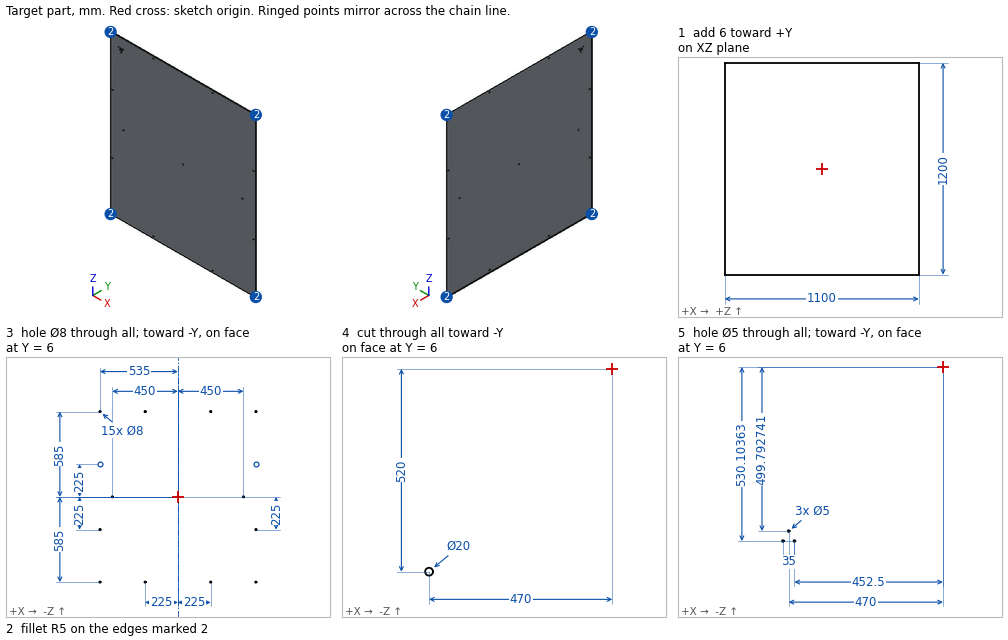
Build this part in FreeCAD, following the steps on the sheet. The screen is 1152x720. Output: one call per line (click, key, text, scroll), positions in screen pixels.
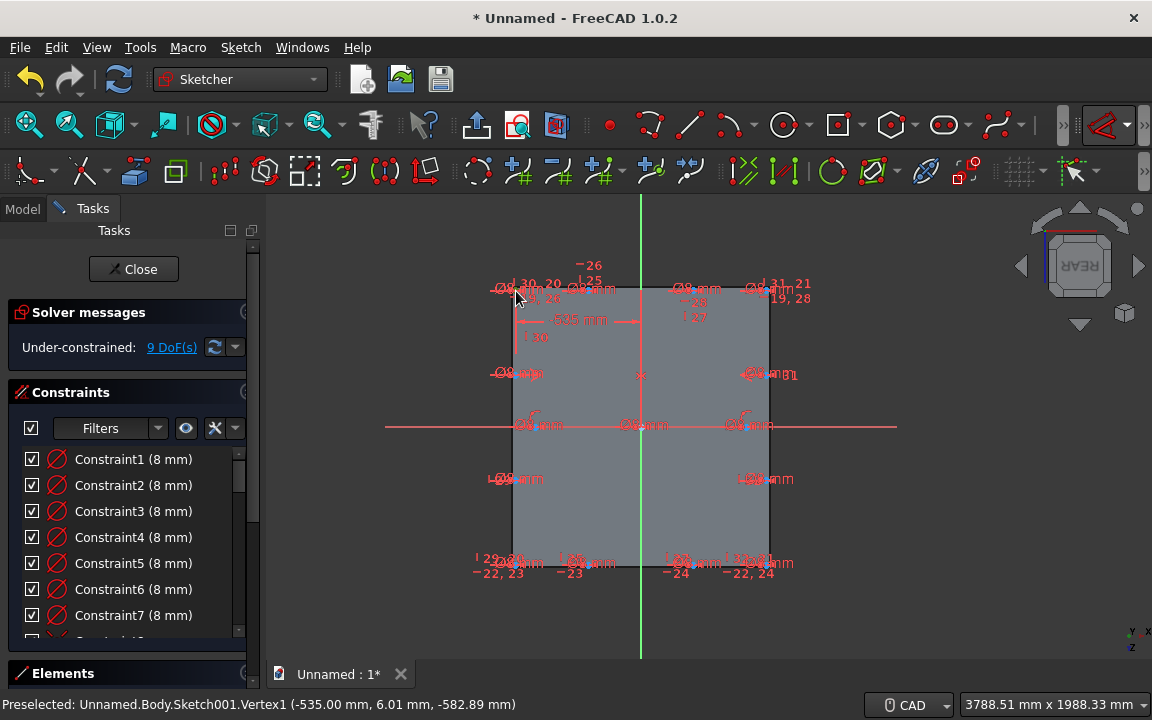
key(i)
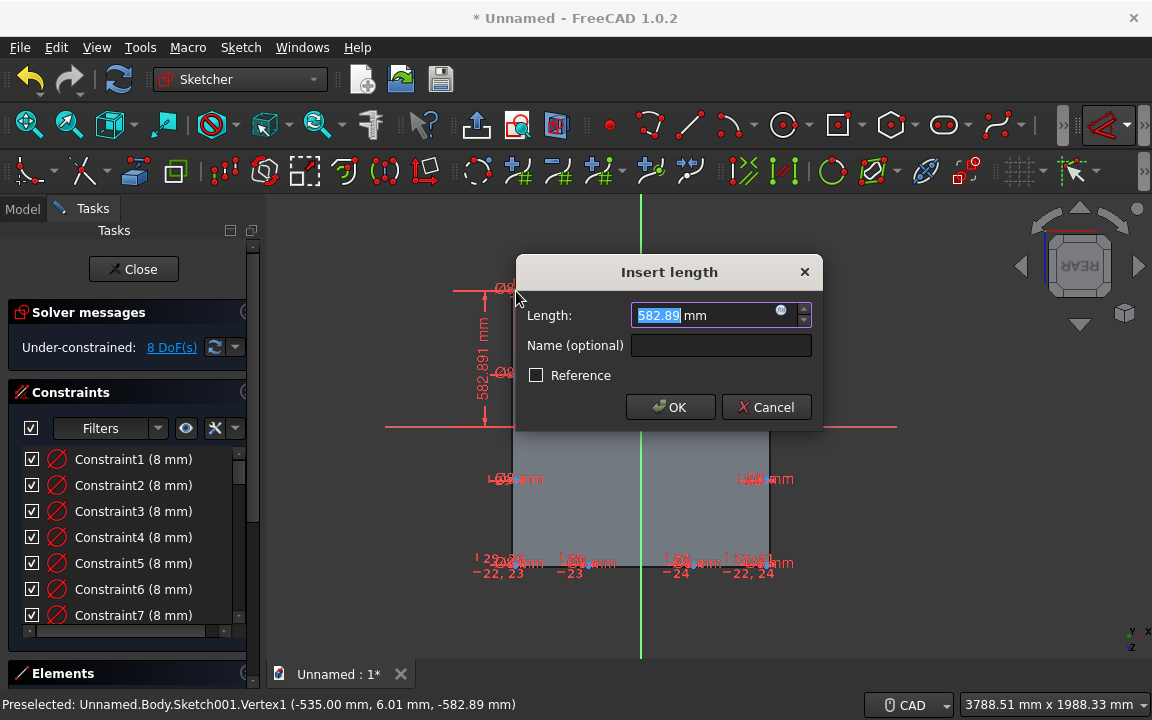
text(585)
key(Return)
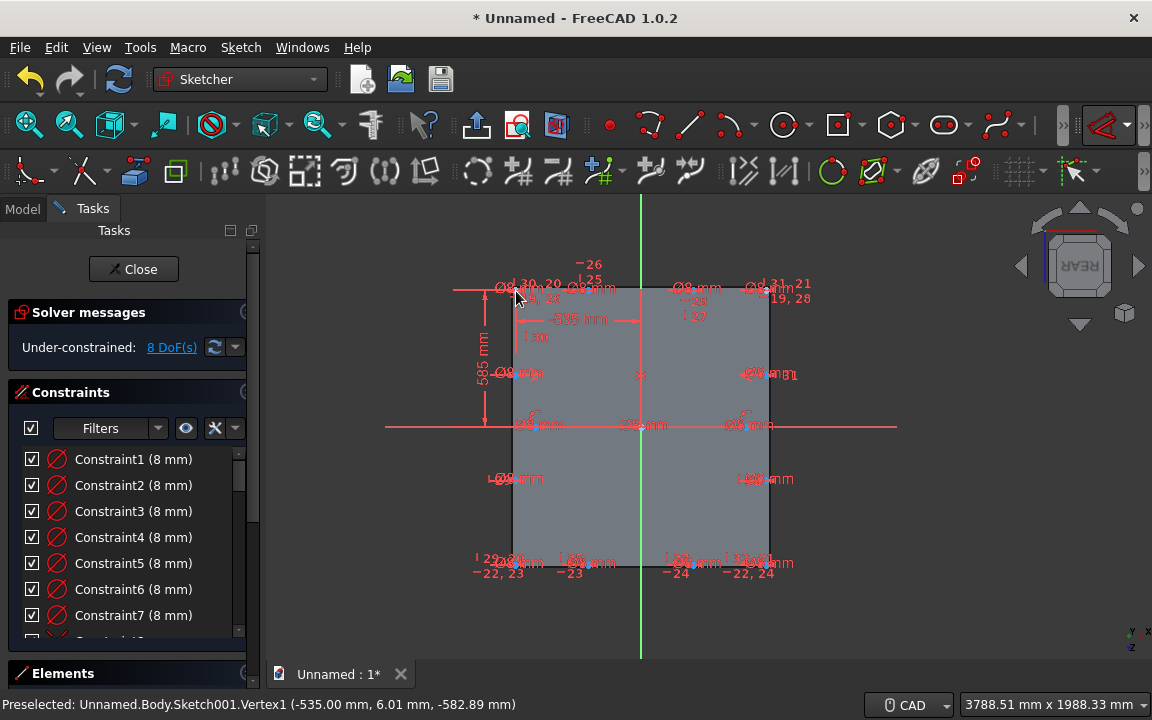
click(516, 565)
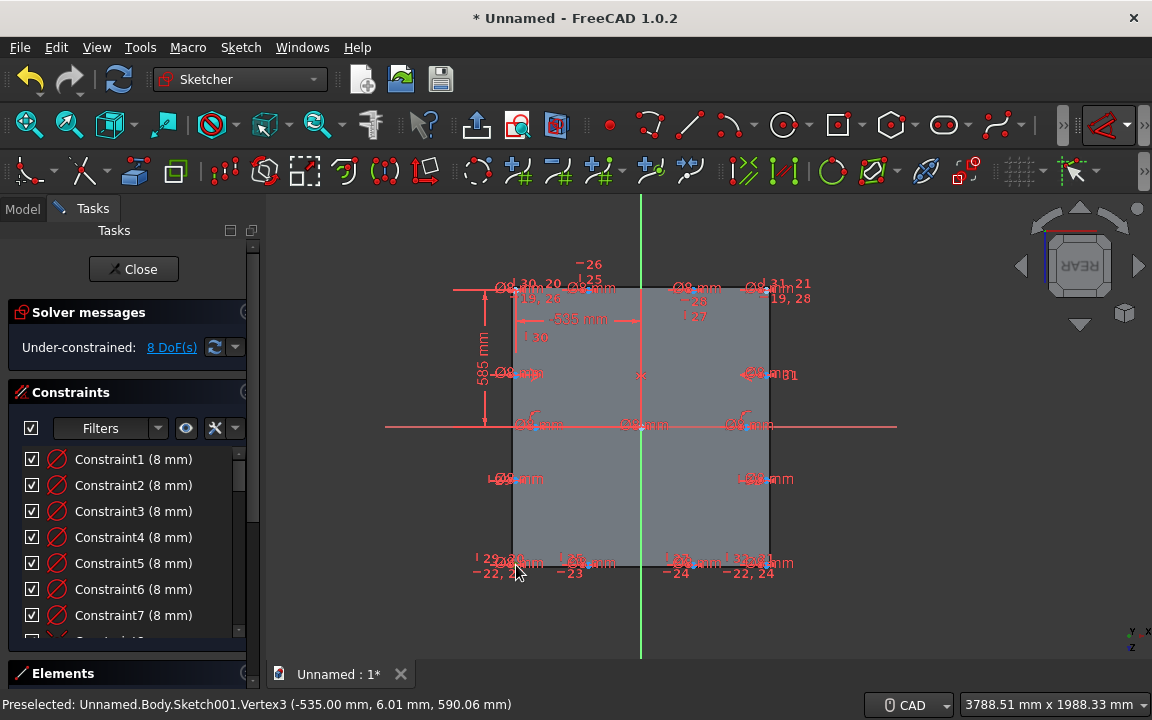
click(1130, 126)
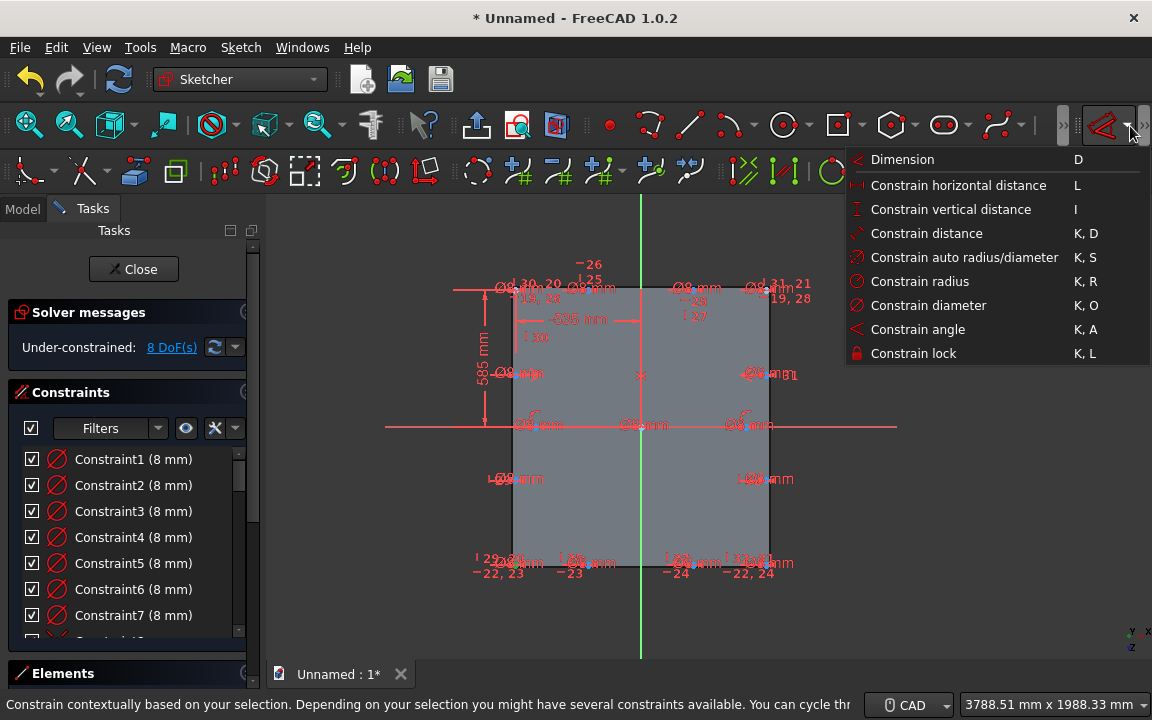
click(998, 209)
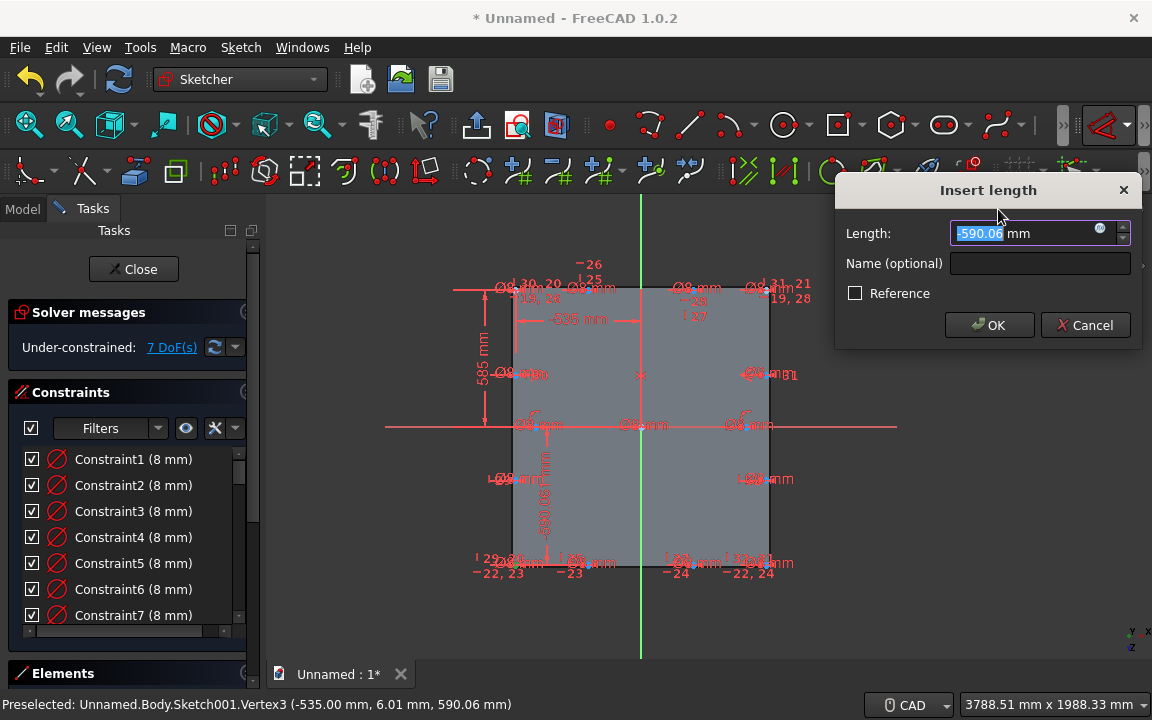
text(-585)
key(Return)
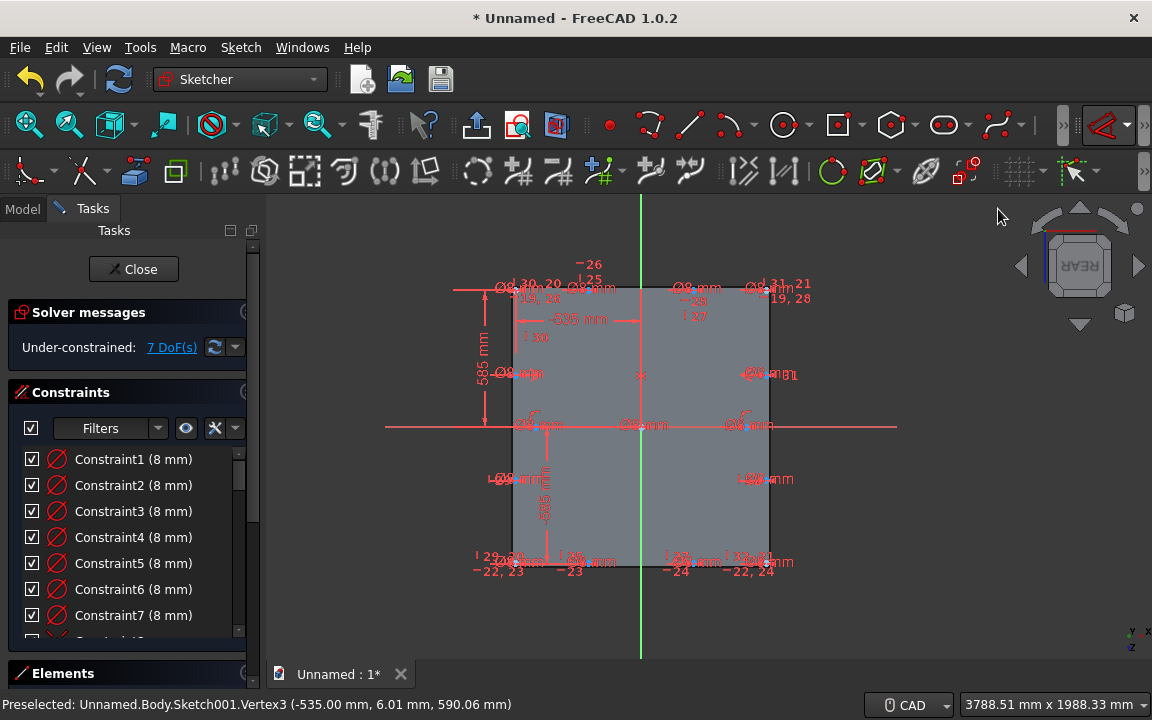
click(588, 564)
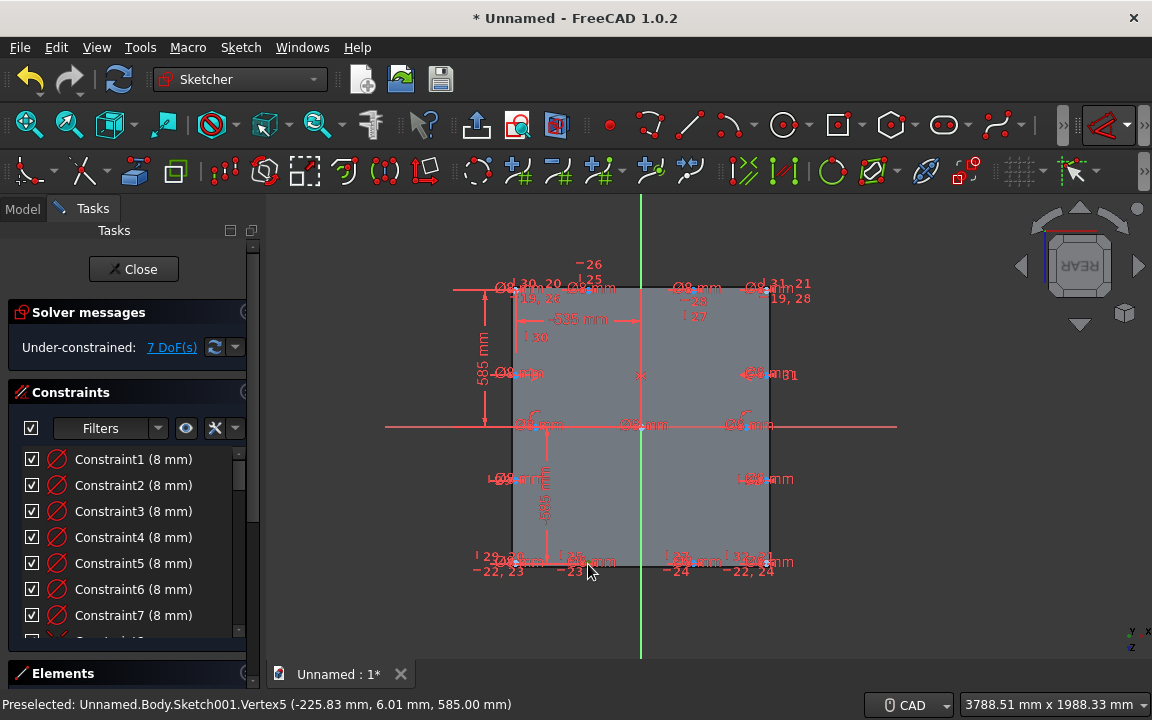
key(l)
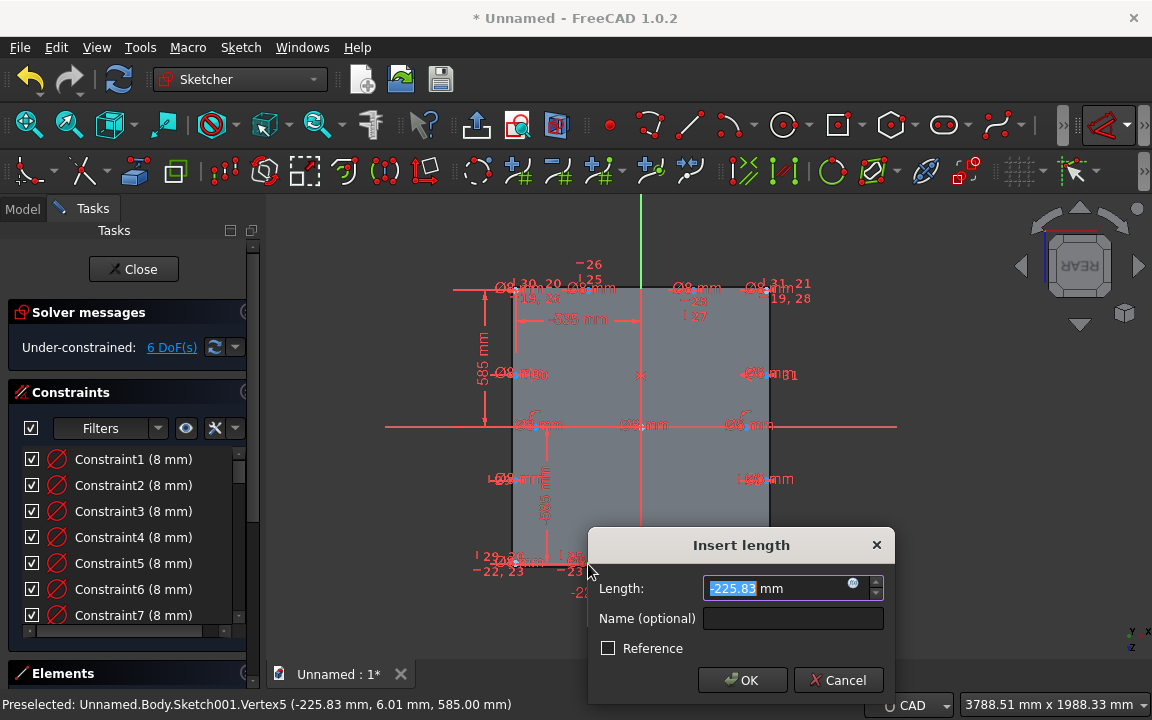
text(-225)
key(Return)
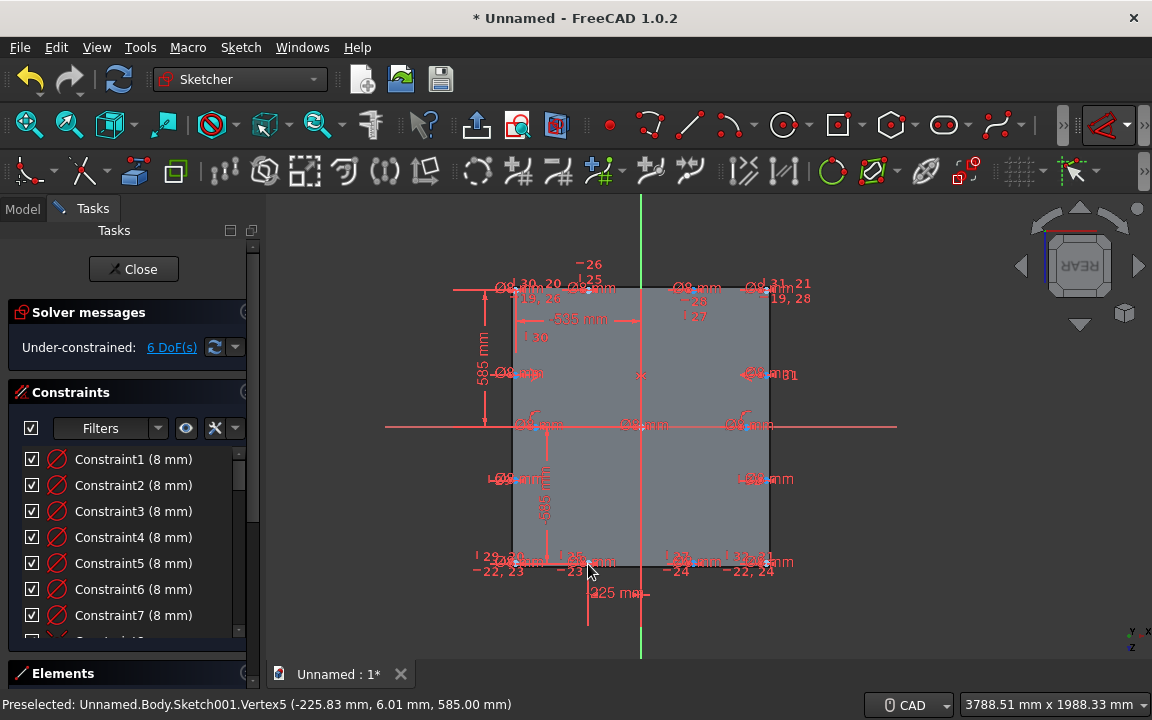
click(694, 564)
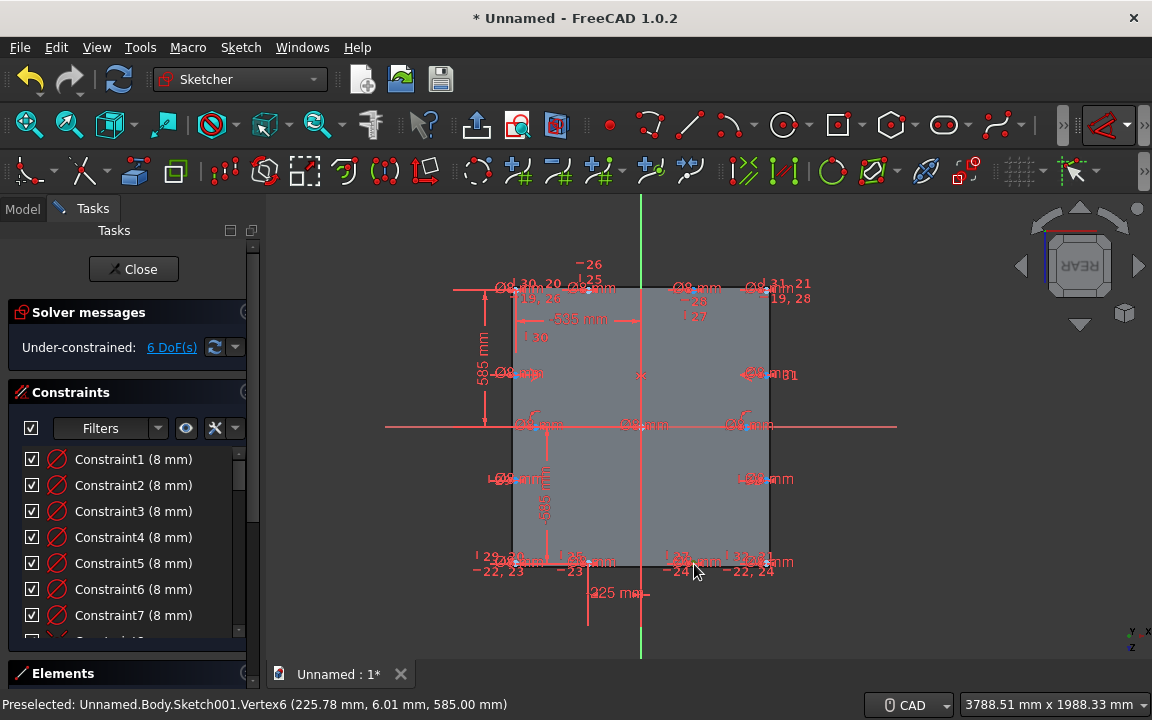
key(l)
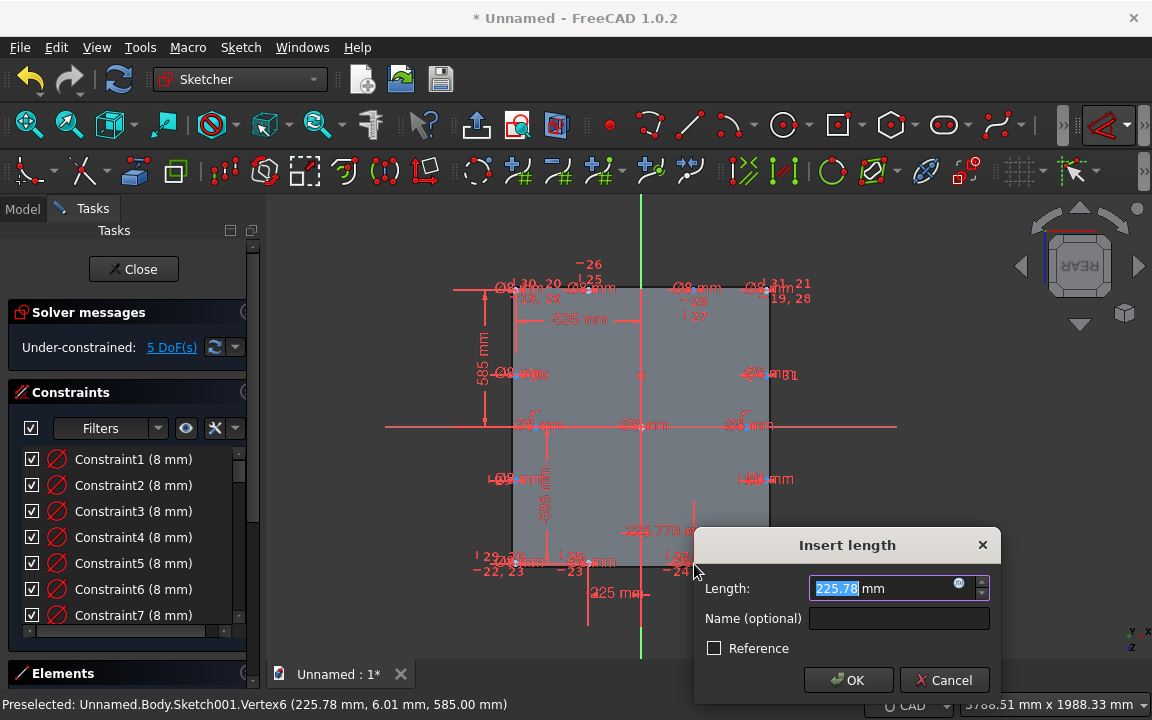
text(225)
key(Return)